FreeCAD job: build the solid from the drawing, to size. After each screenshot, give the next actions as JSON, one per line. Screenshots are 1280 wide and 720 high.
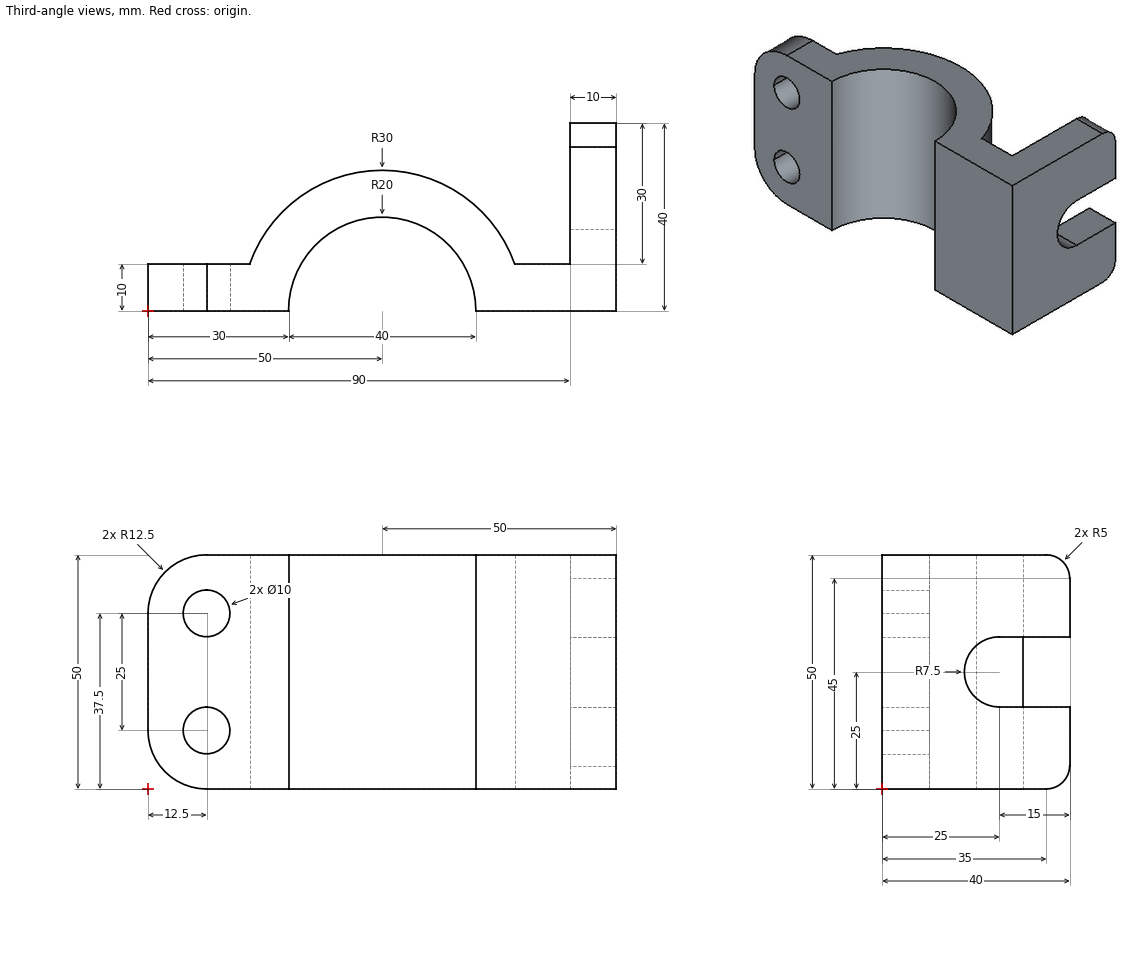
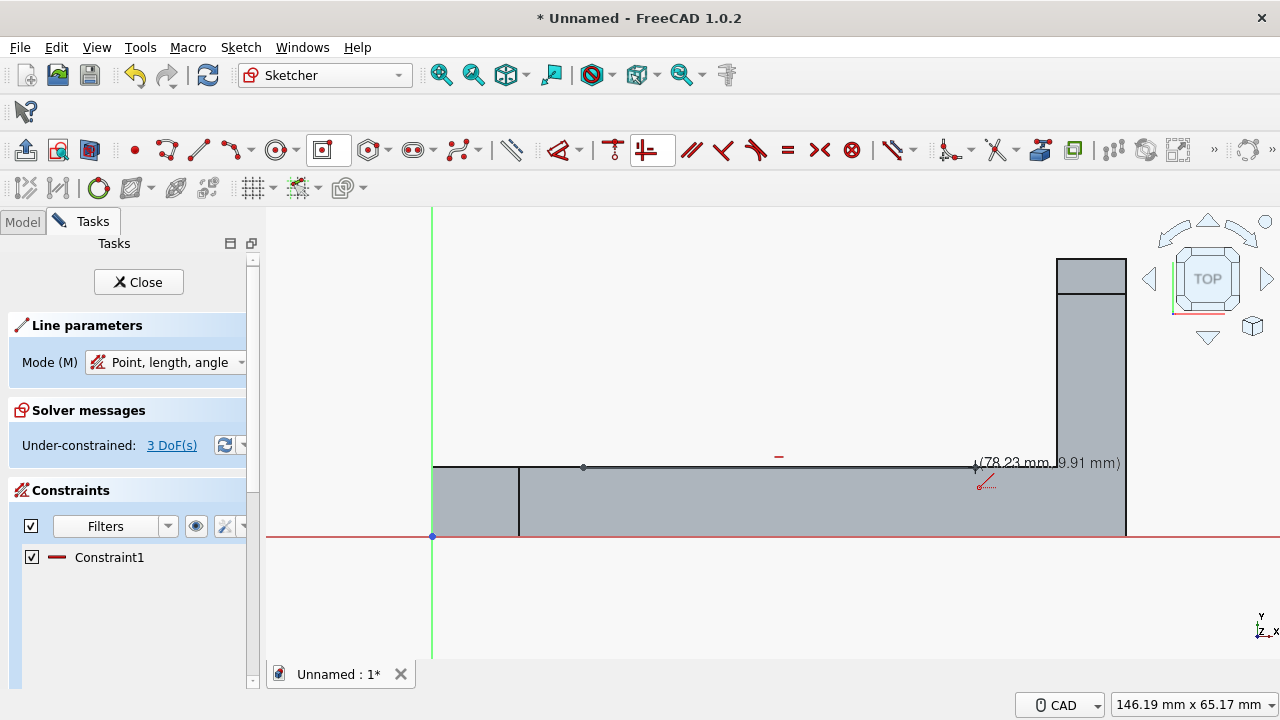
{"action": "left_click", "coordinate": [232, 150]}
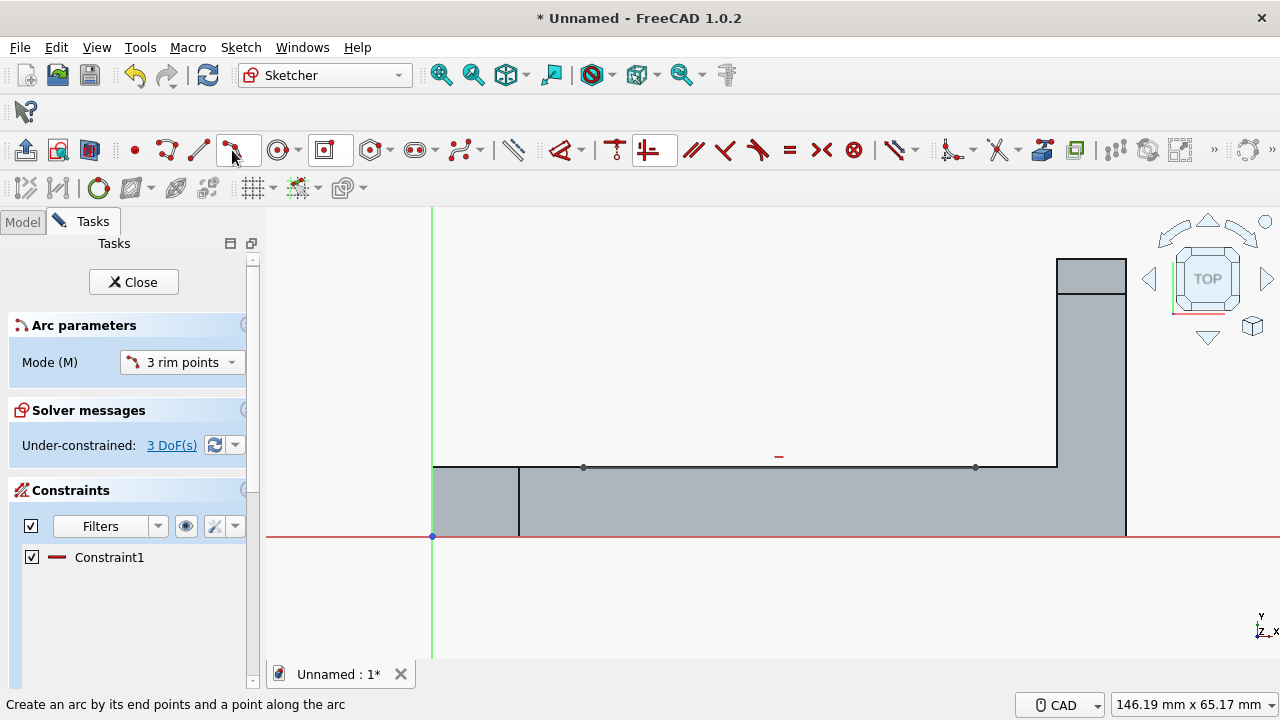
{"action": "left_click", "coordinate": [975, 468]}
{"action": "left_click", "coordinate": [583, 468]}
{"action": "left_click", "coordinate": [779, 329]}
{"action": "key", "text": "Escape"}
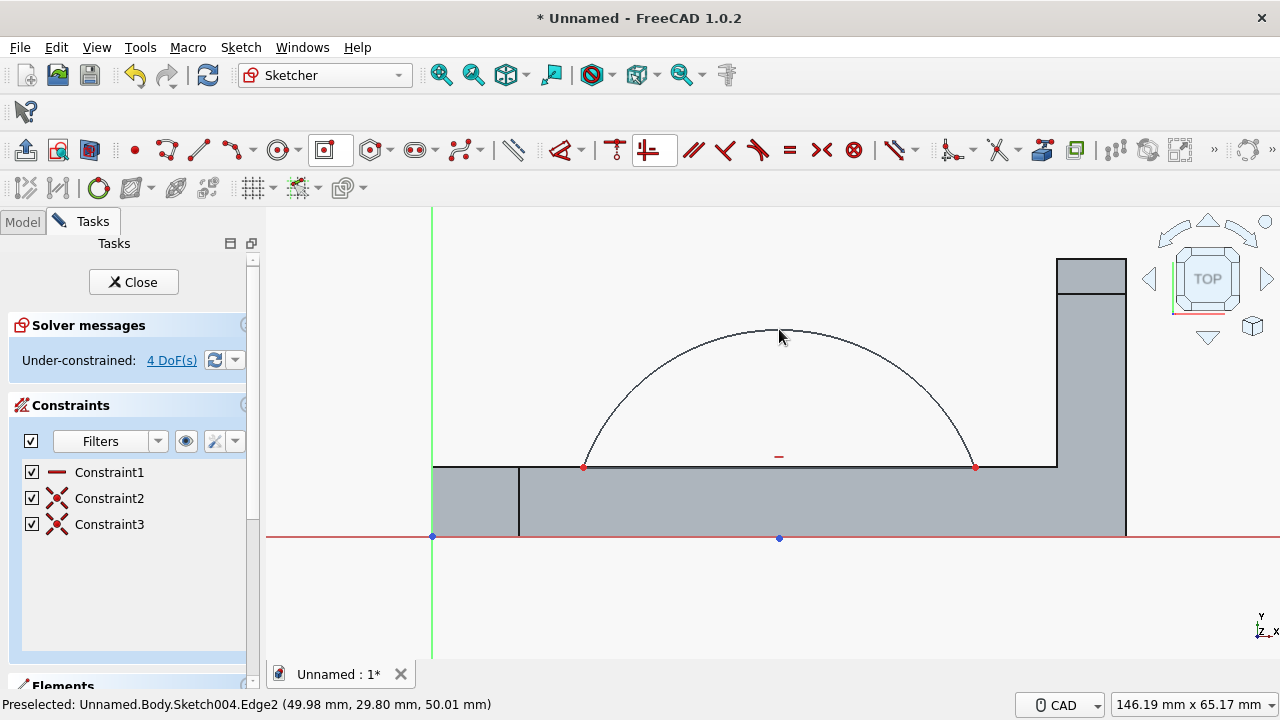
{"action": "left_click", "coordinate": [779, 538]}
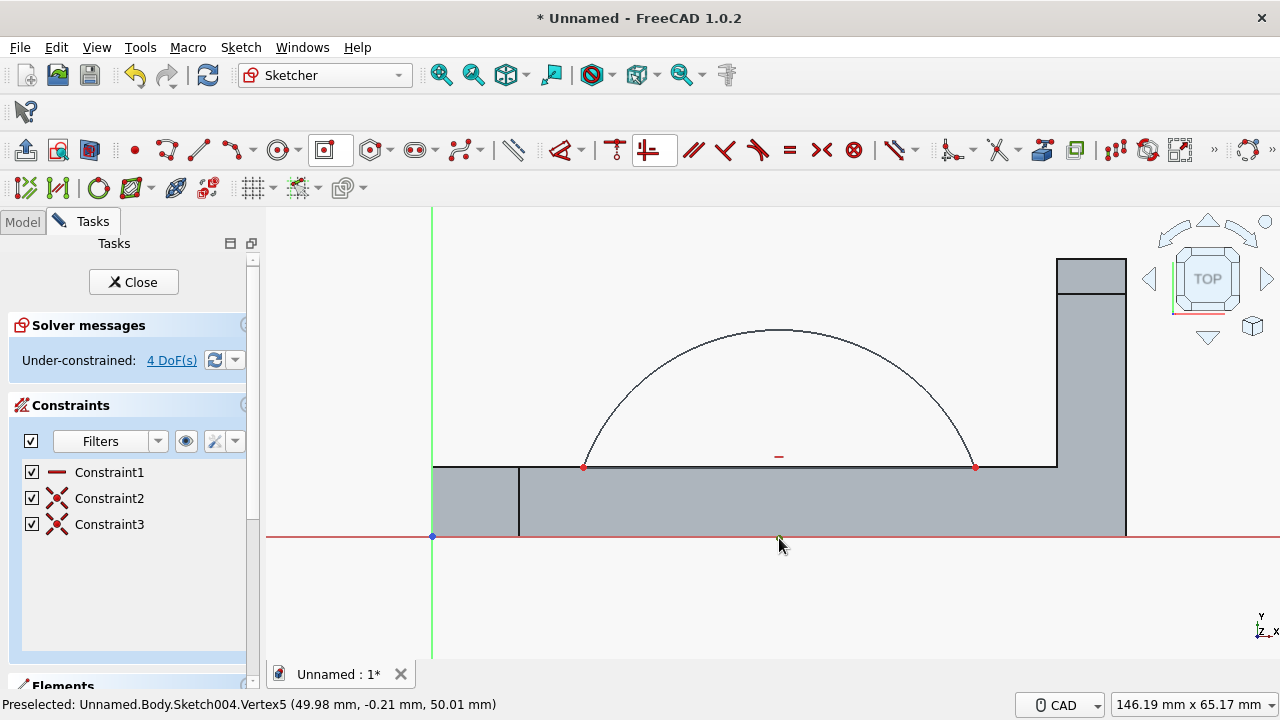
{"action": "left_click", "coordinate": [353, 537]}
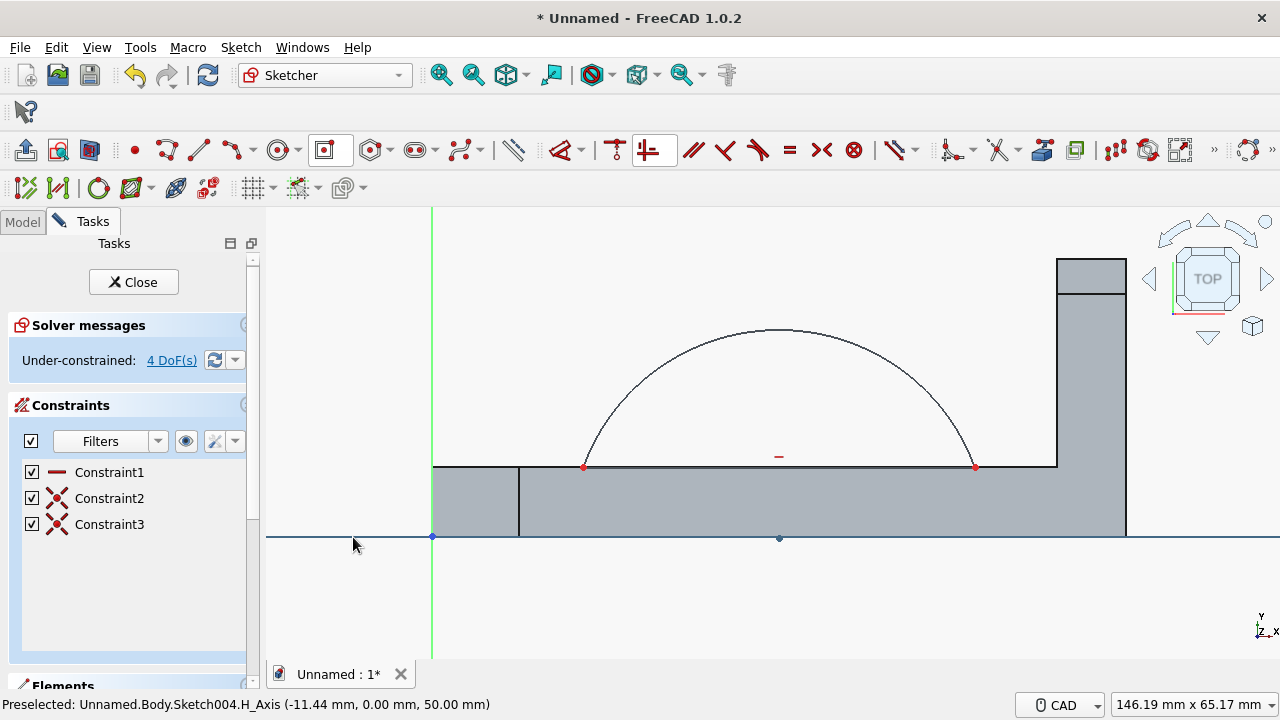
{"action": "left_click", "coordinate": [616, 150]}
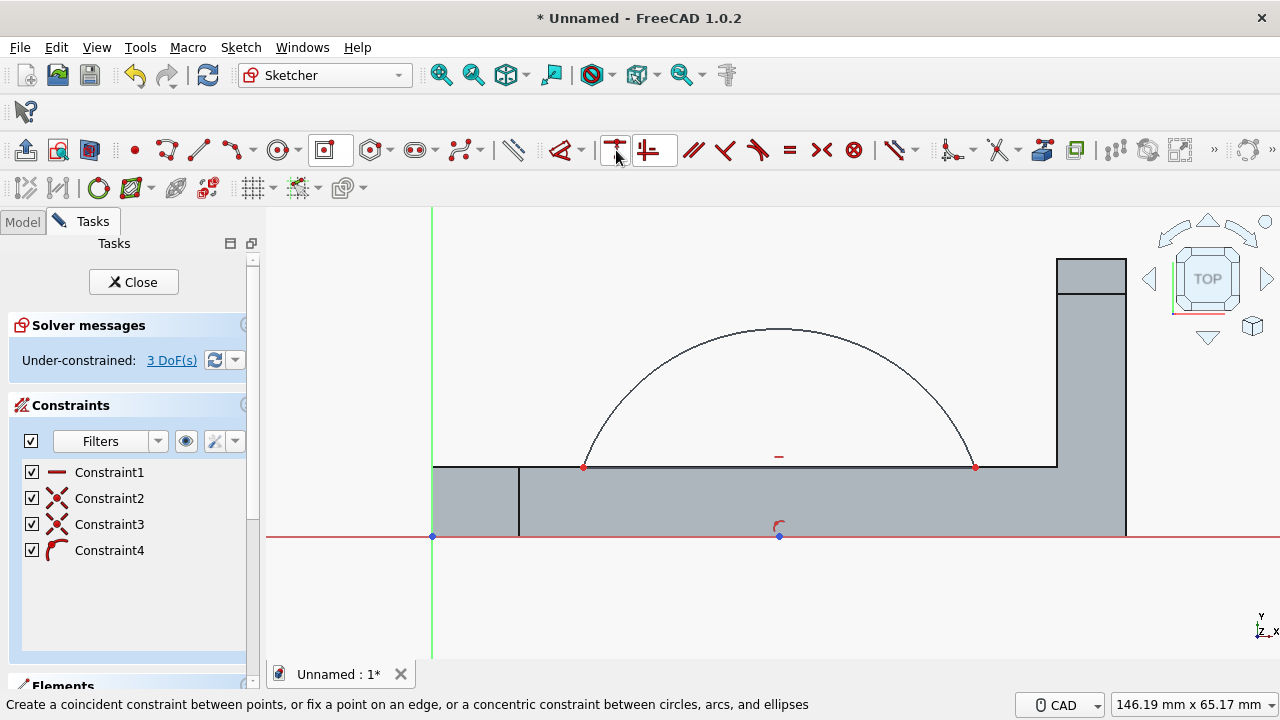
{"action": "left_click", "coordinate": [560, 150]}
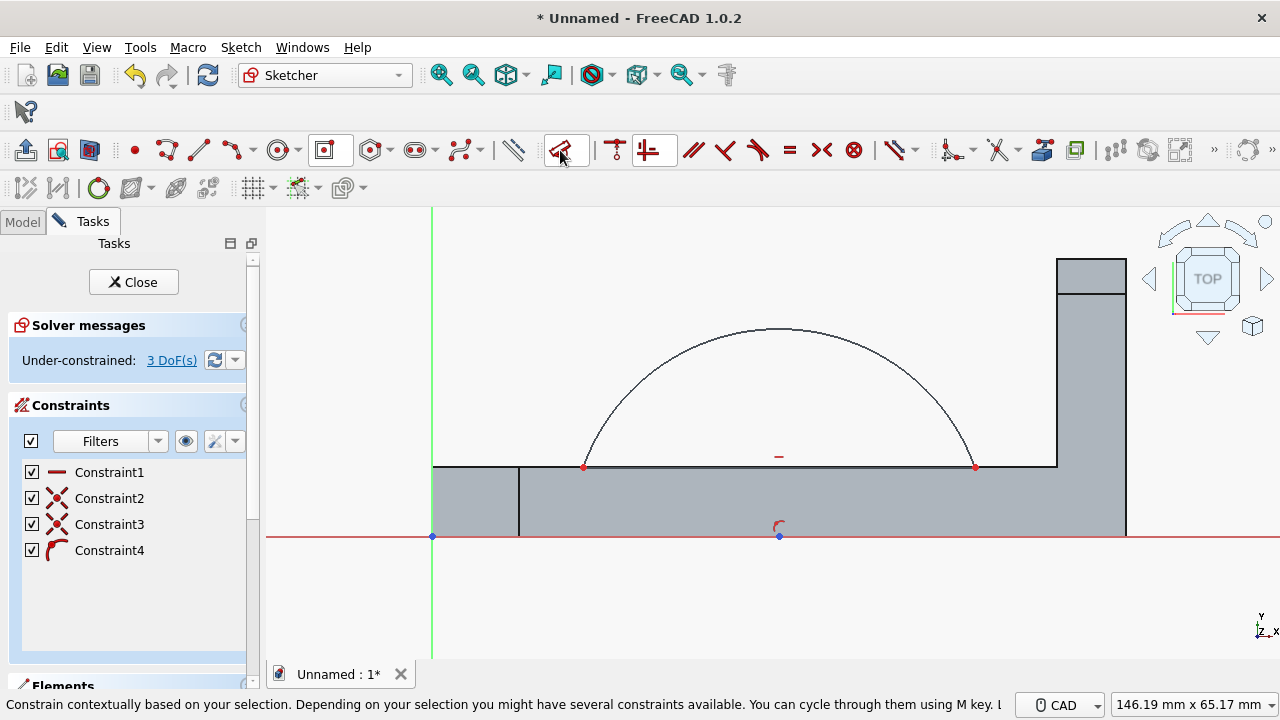
{"action": "left_click", "coordinate": [877, 354]}
{"action": "left_click", "coordinate": [892, 326]}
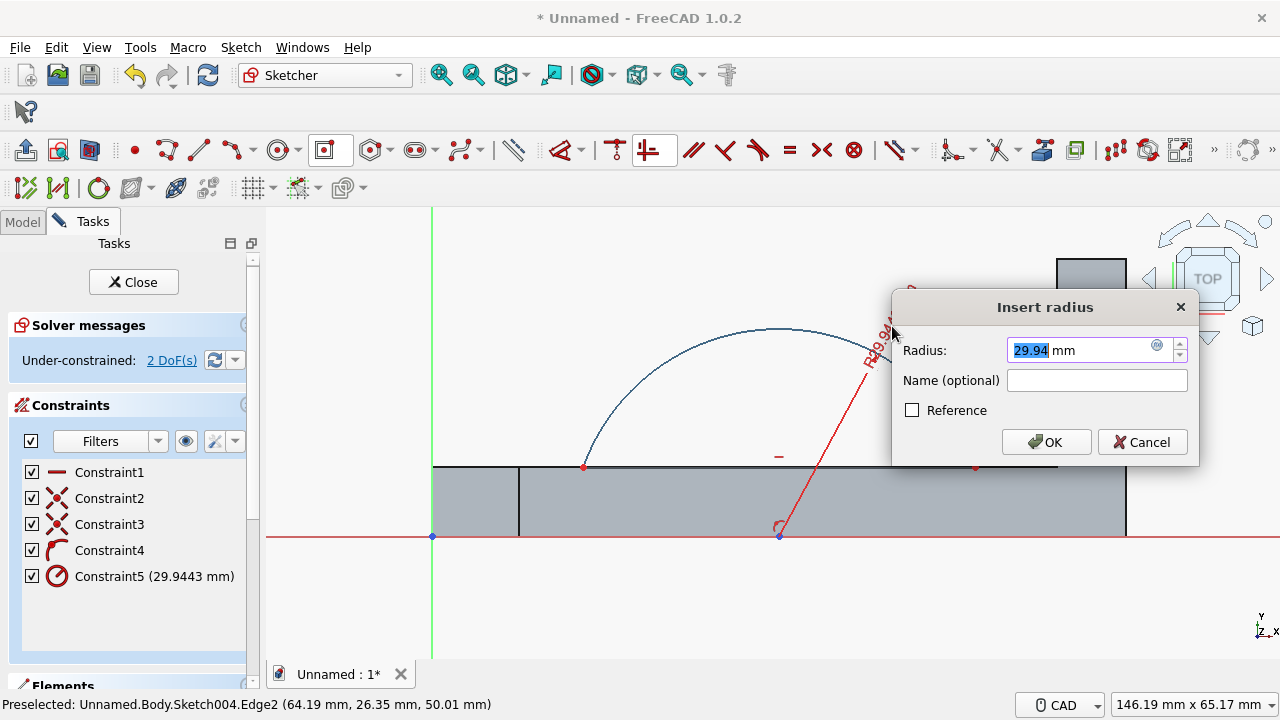
{"action": "type", "text": "30"}
{"action": "key", "text": "Return"}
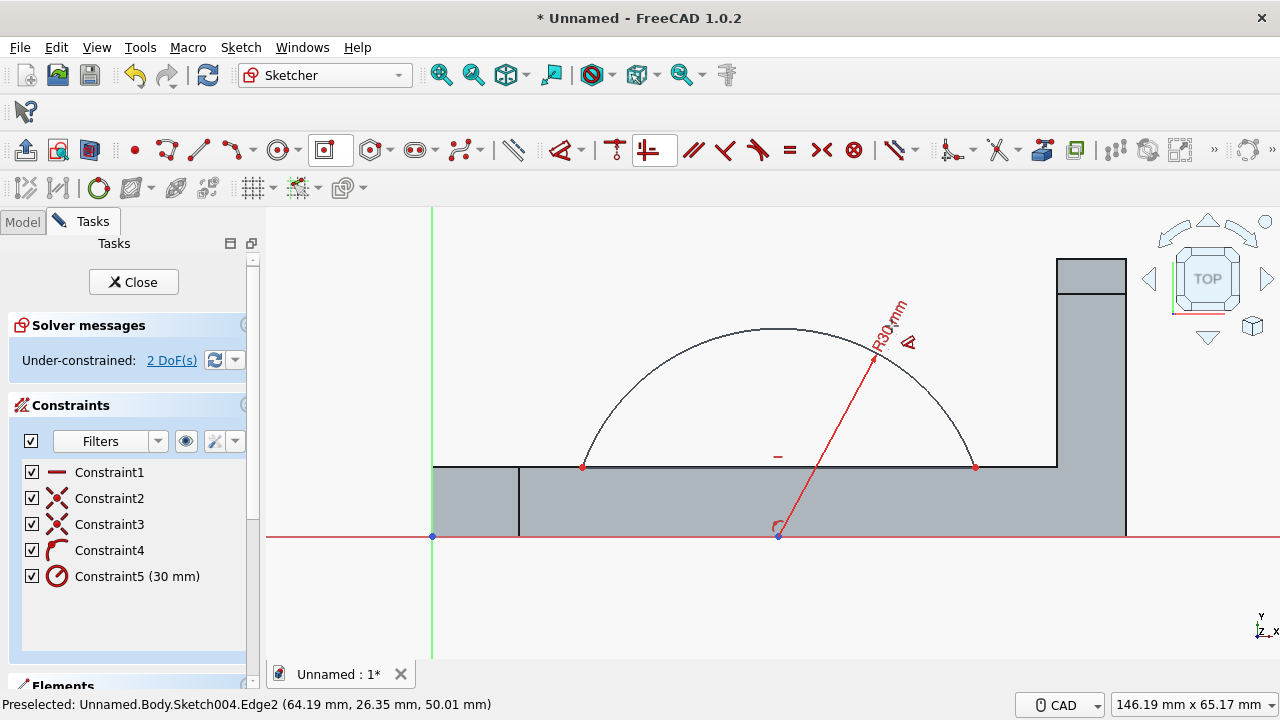
{"action": "left_click", "coordinate": [582, 468]}
{"action": "left_click", "coordinate": [398, 502]}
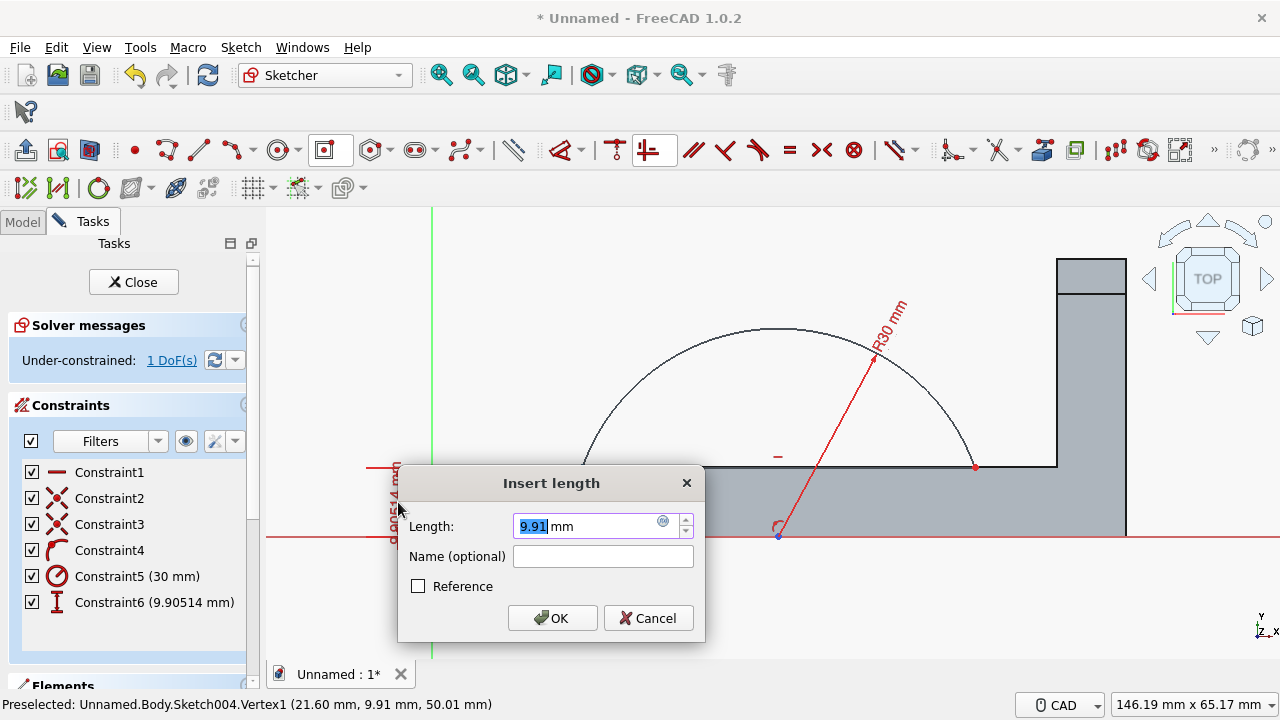
{"action": "type", "text": "10"}
{"action": "key", "text": "Return"}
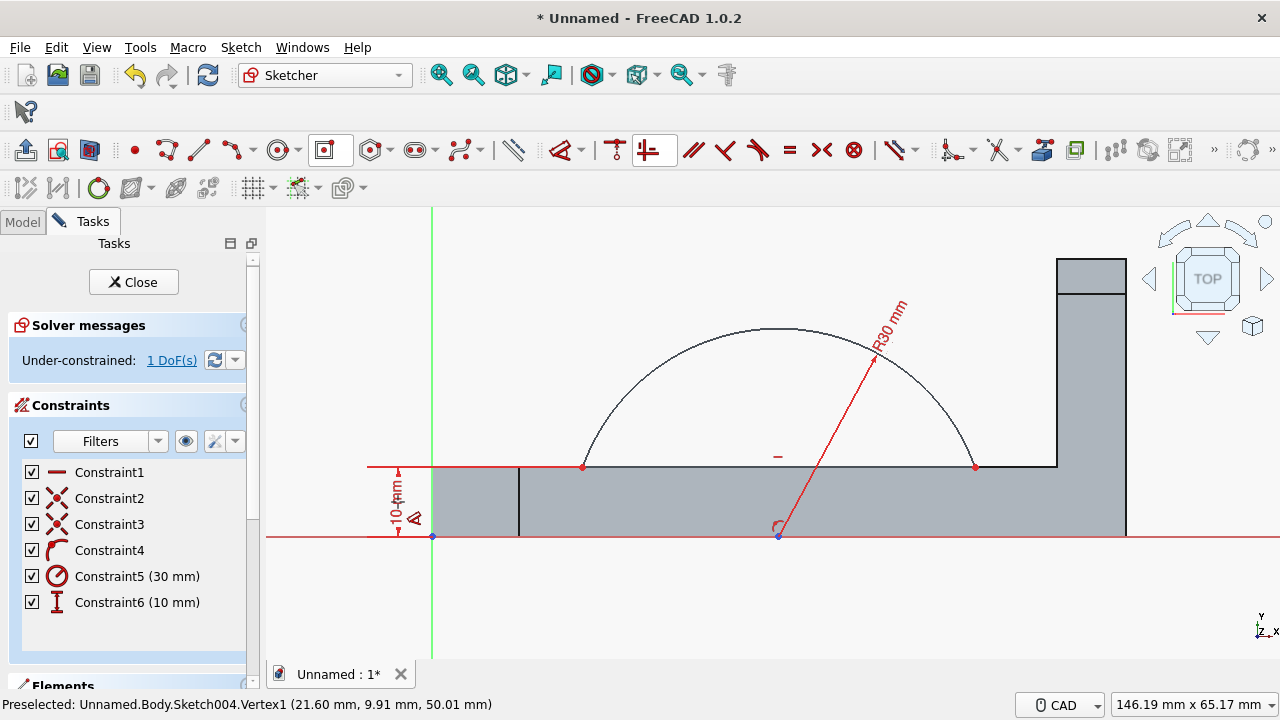
{"action": "left_click", "coordinate": [779, 537]}
{"action": "left_click", "coordinate": [606, 571]}